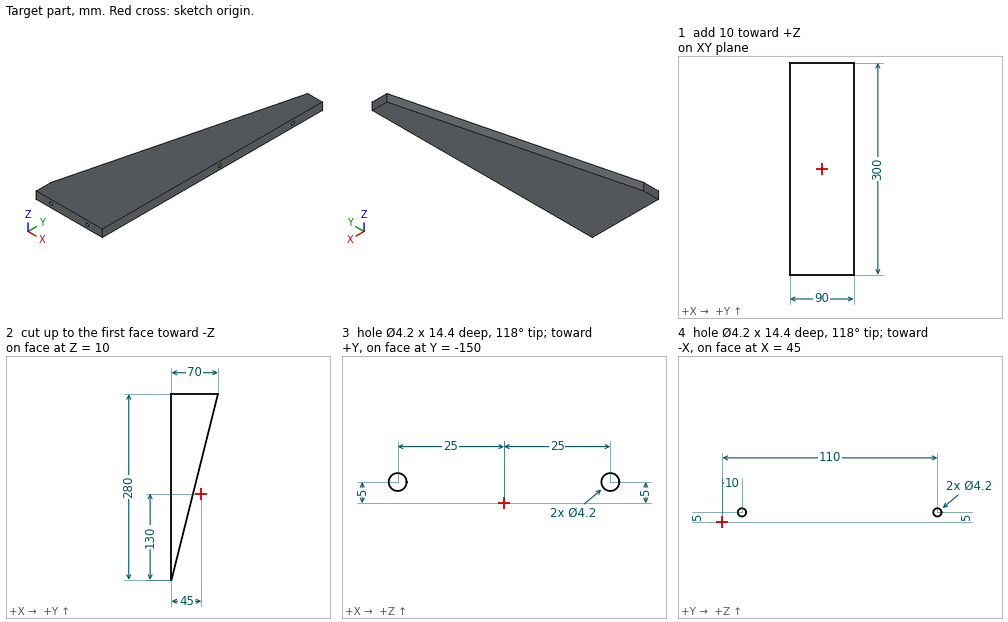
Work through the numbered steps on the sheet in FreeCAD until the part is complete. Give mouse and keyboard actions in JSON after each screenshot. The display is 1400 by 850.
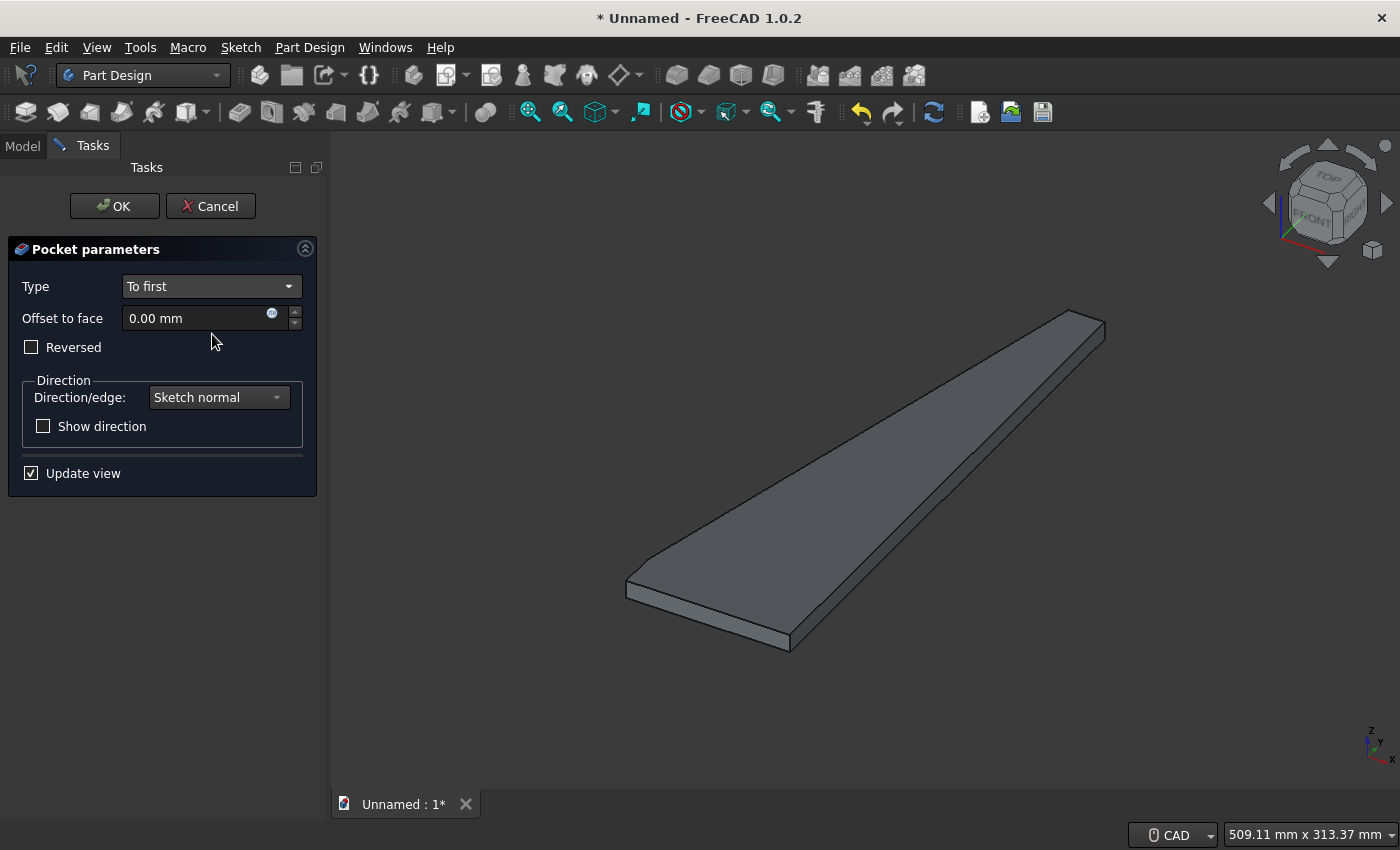
{"action": "left_click", "coordinate": [115, 206]}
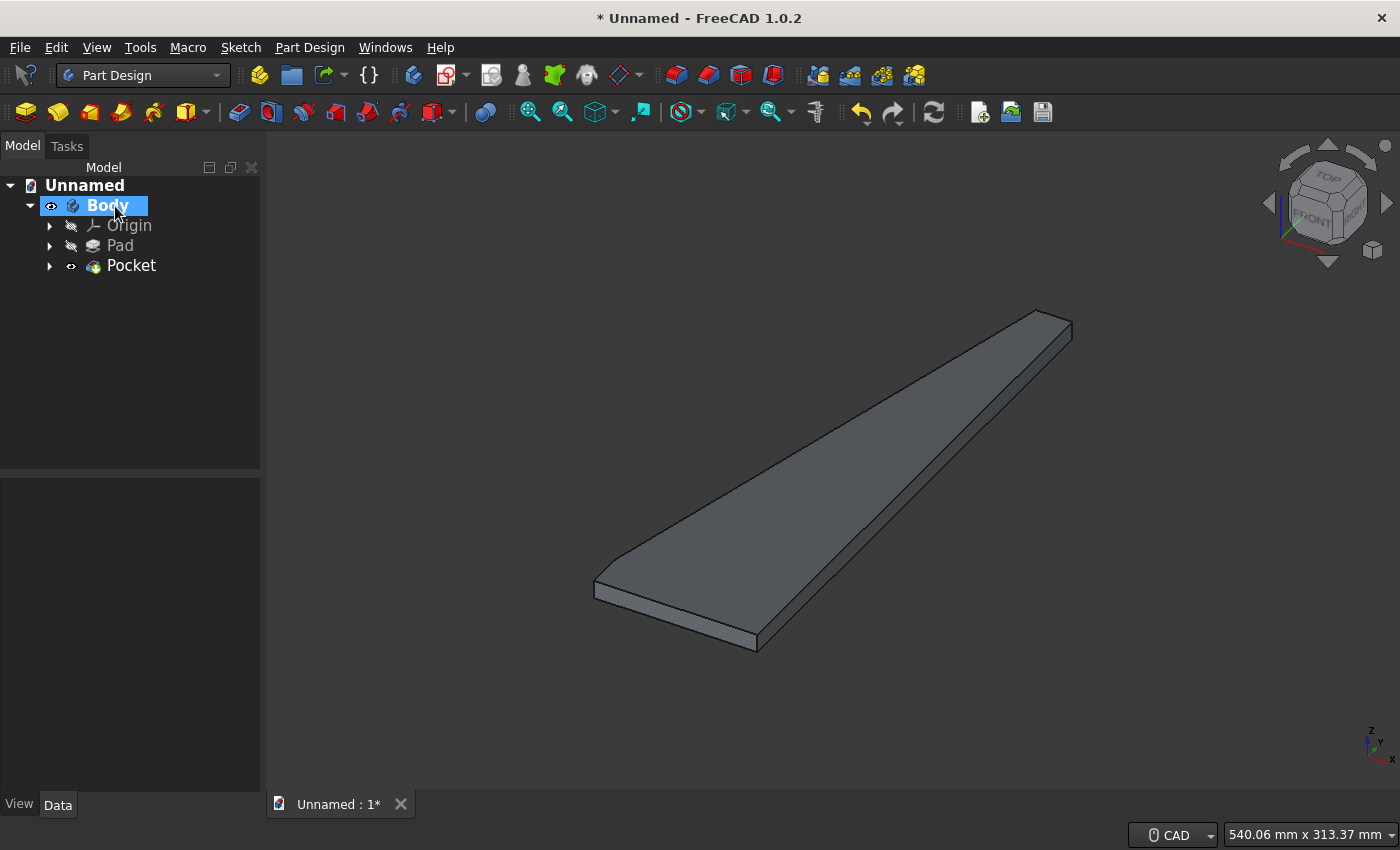
{"action": "key", "text": "0"}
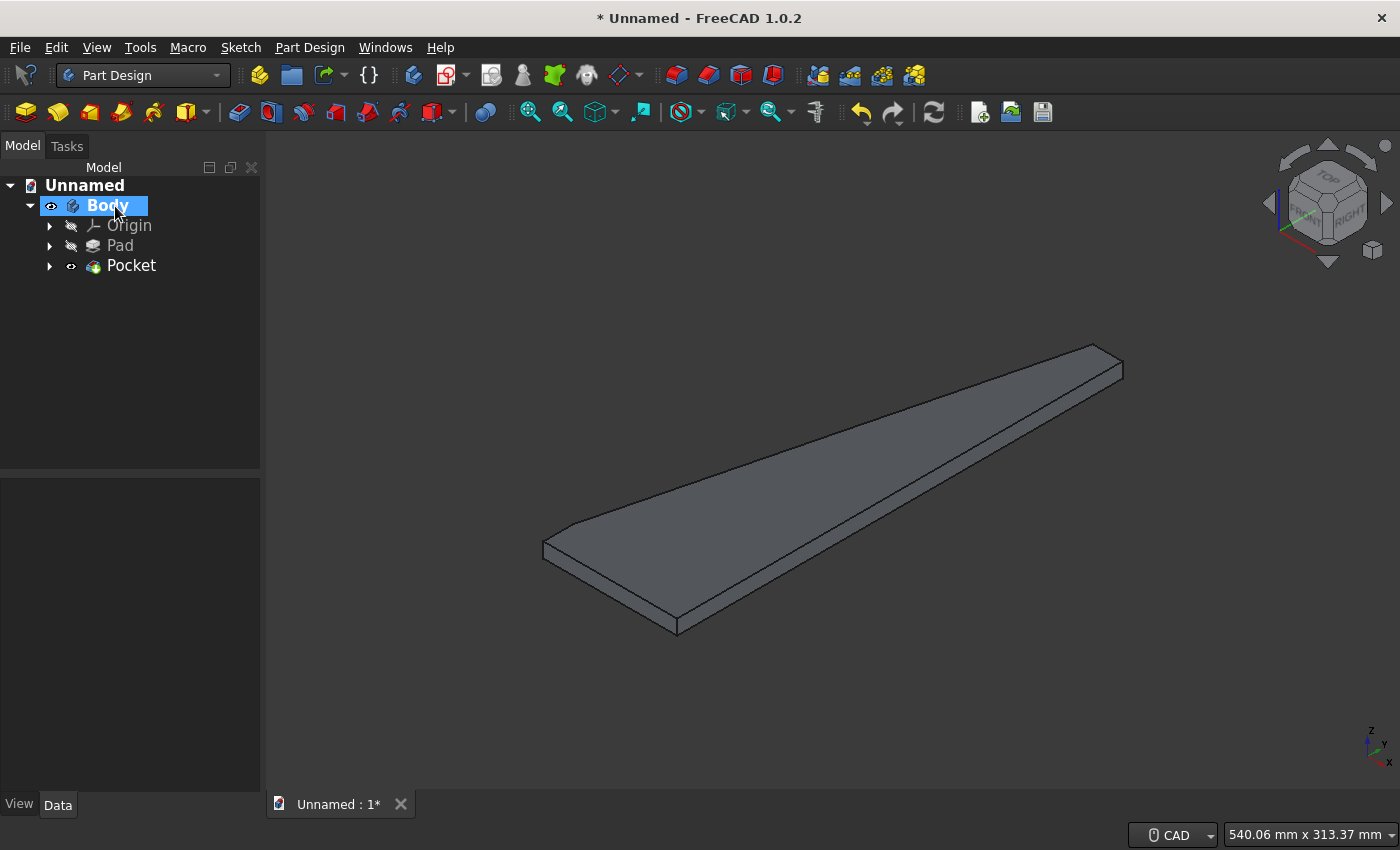
{"action": "key", "text": "1"}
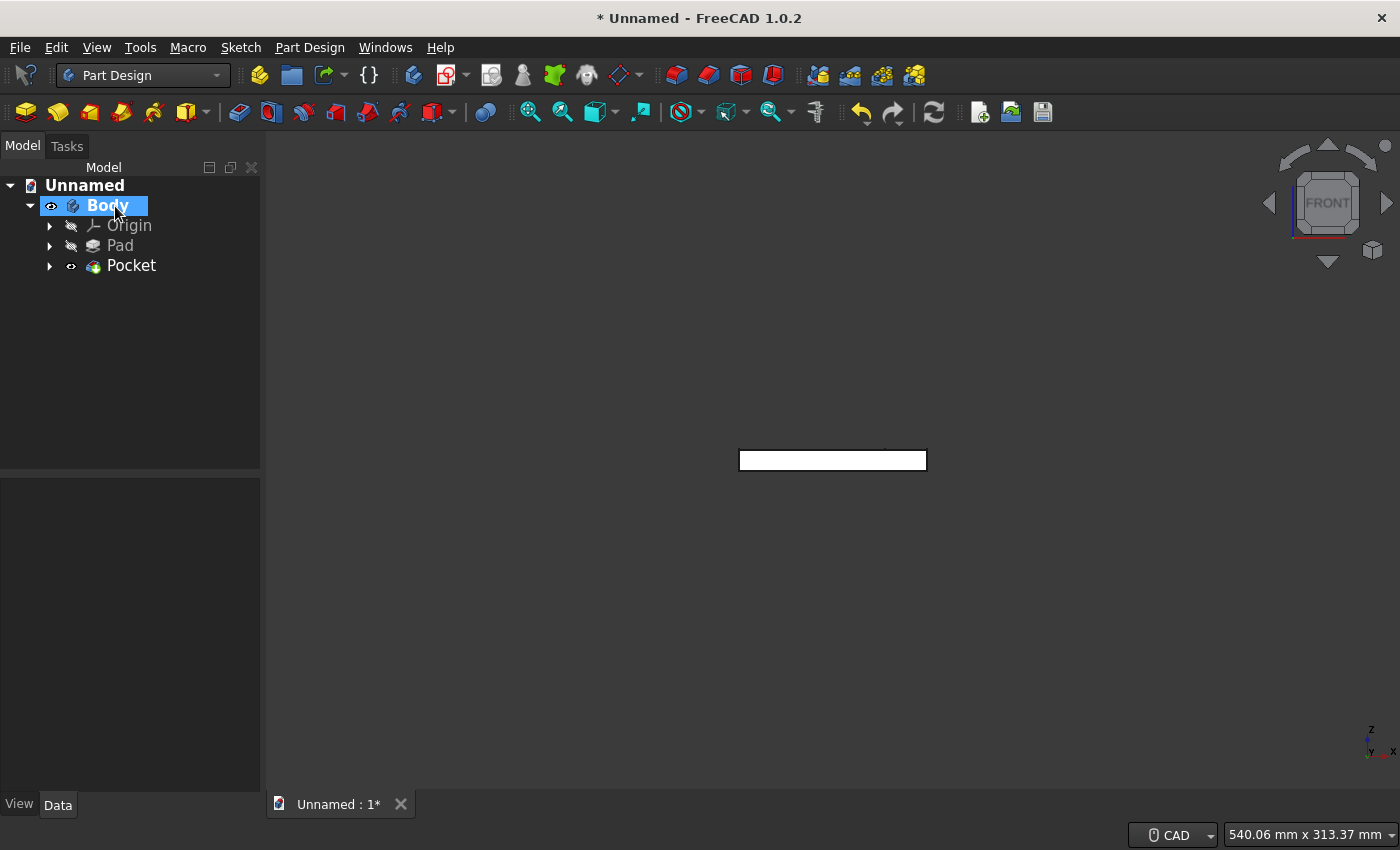
{"action": "key", "text": "v f"}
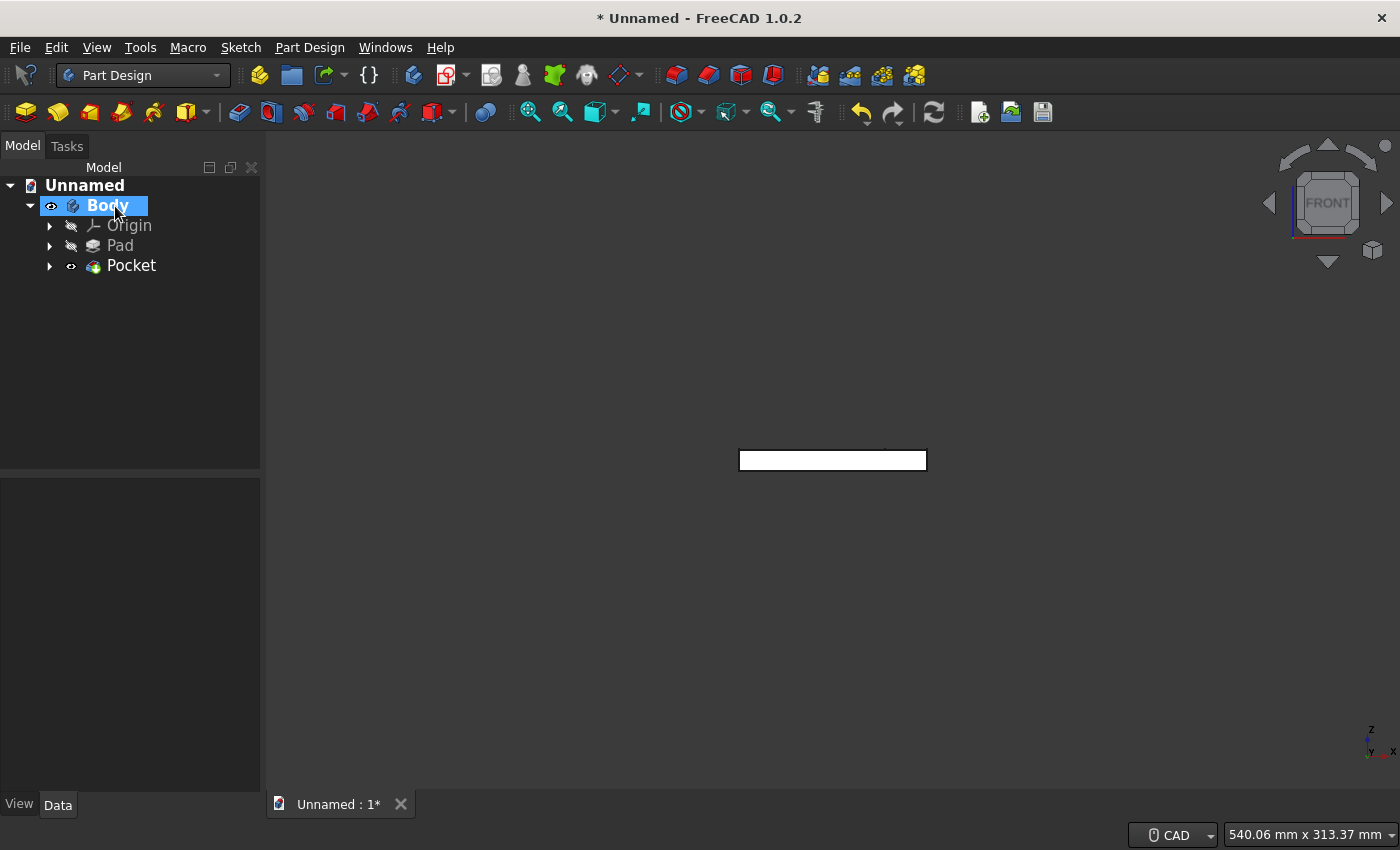
{"action": "left_click", "coordinate": [914, 459]}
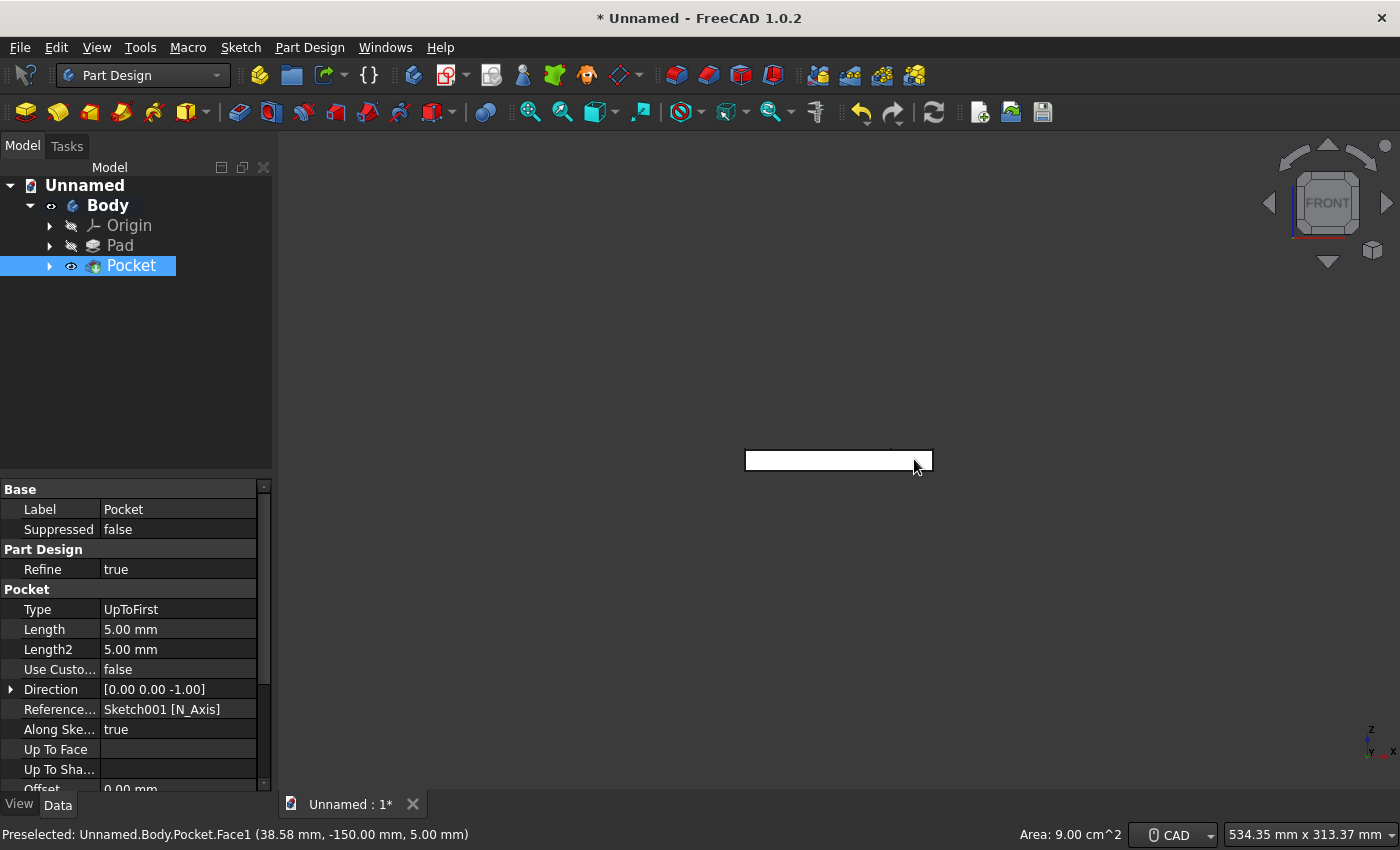
{"action": "left_click", "coordinate": [446, 76]}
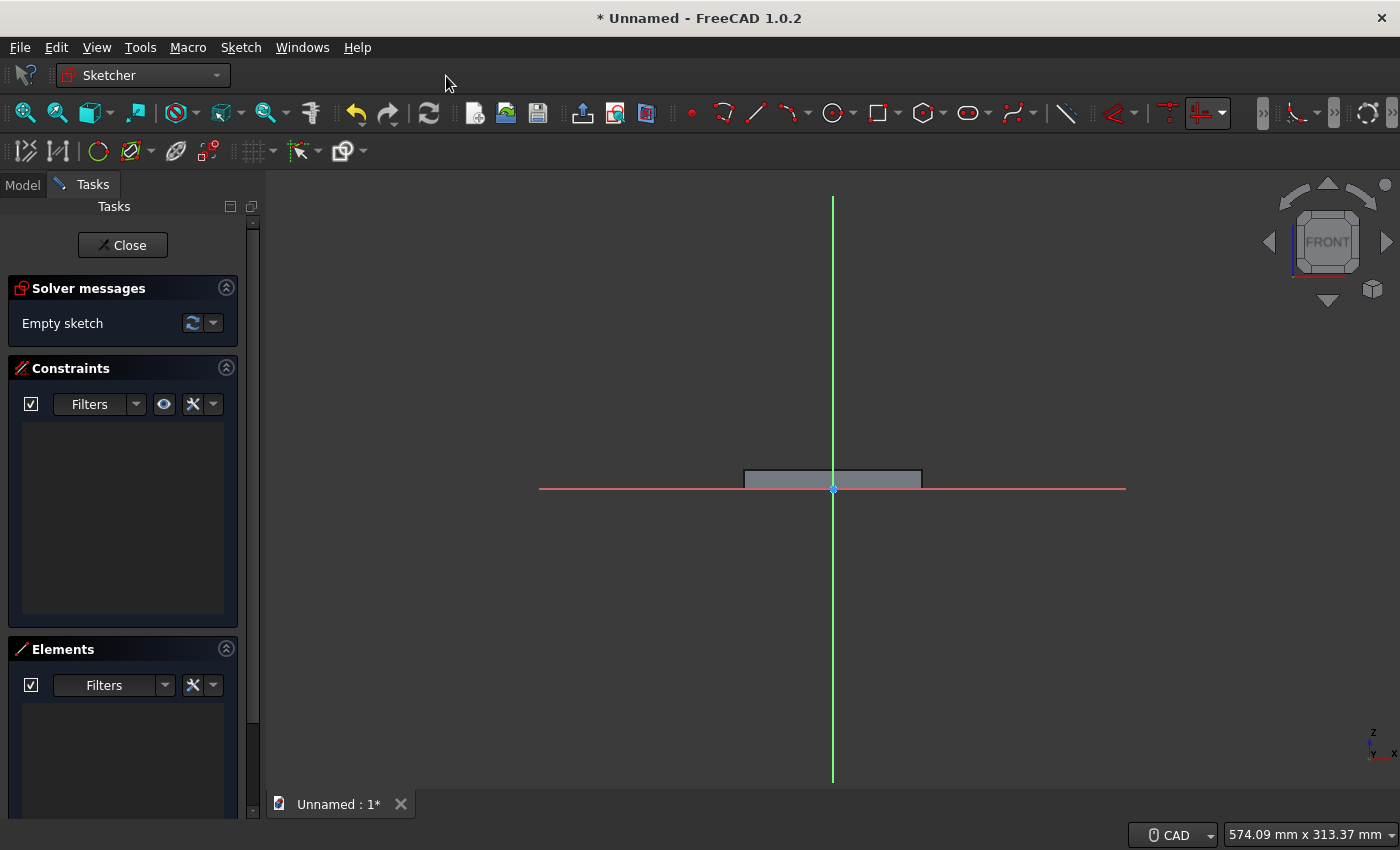
{"action": "scroll", "coordinate": [847, 483], "scroll_direction": "up", "scroll_amount": 9}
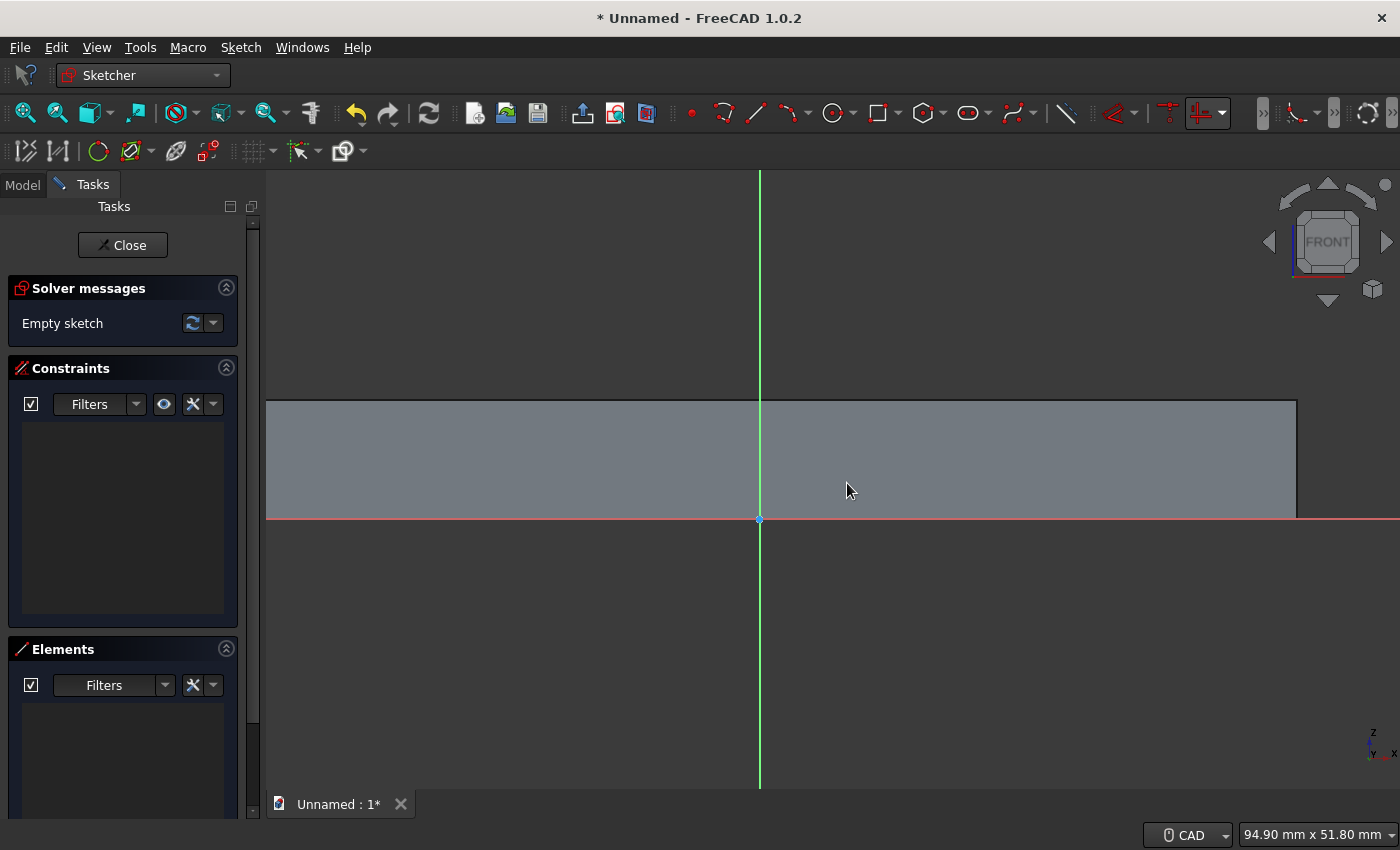
{"action": "left_click", "coordinate": [834, 114]}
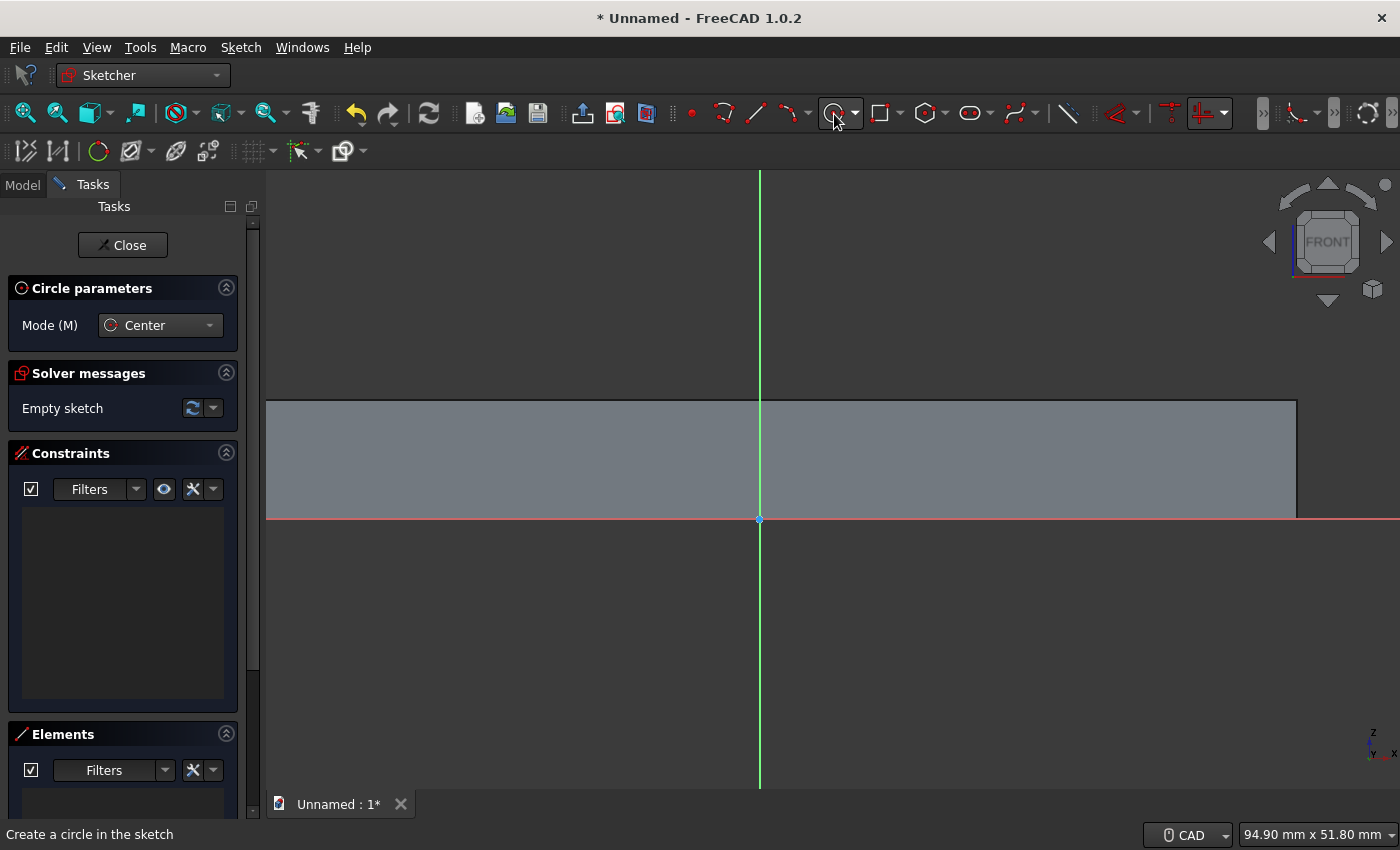
{"action": "left_click", "coordinate": [1058, 459]}
{"action": "left_click", "coordinate": [1076, 442]}